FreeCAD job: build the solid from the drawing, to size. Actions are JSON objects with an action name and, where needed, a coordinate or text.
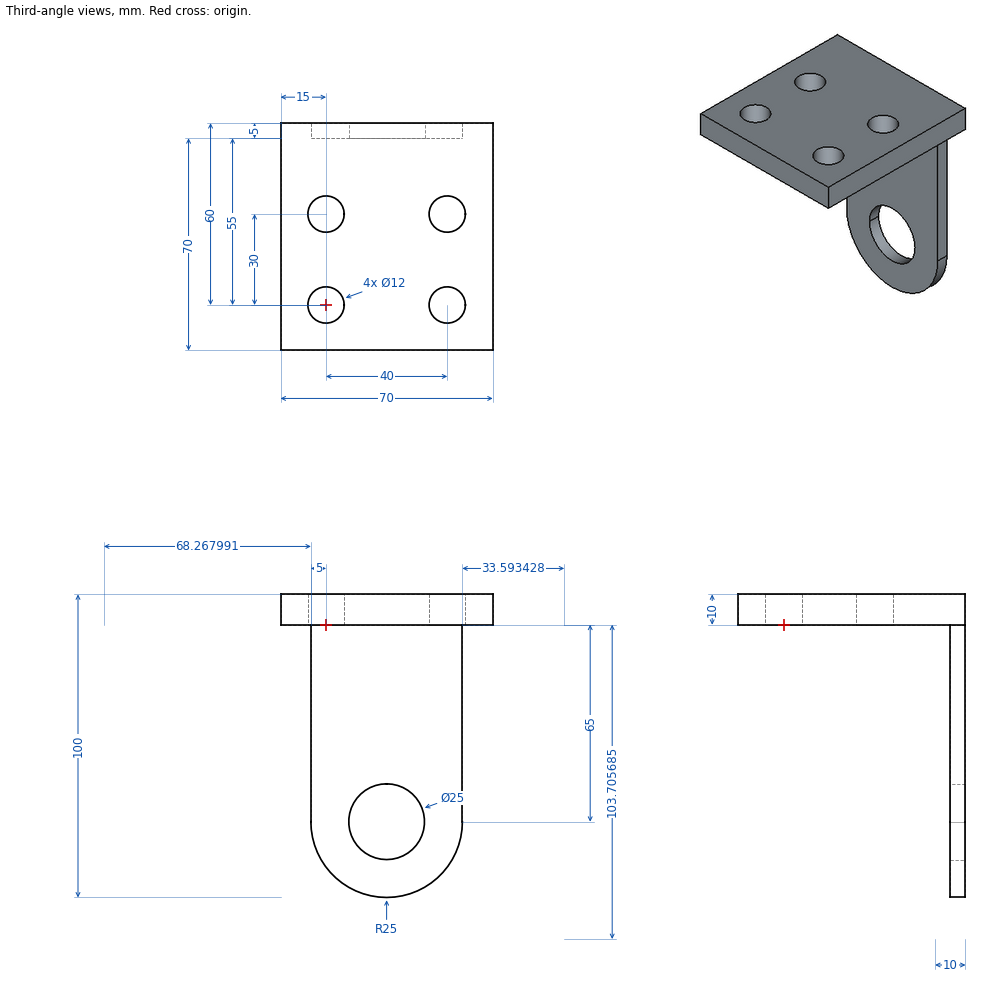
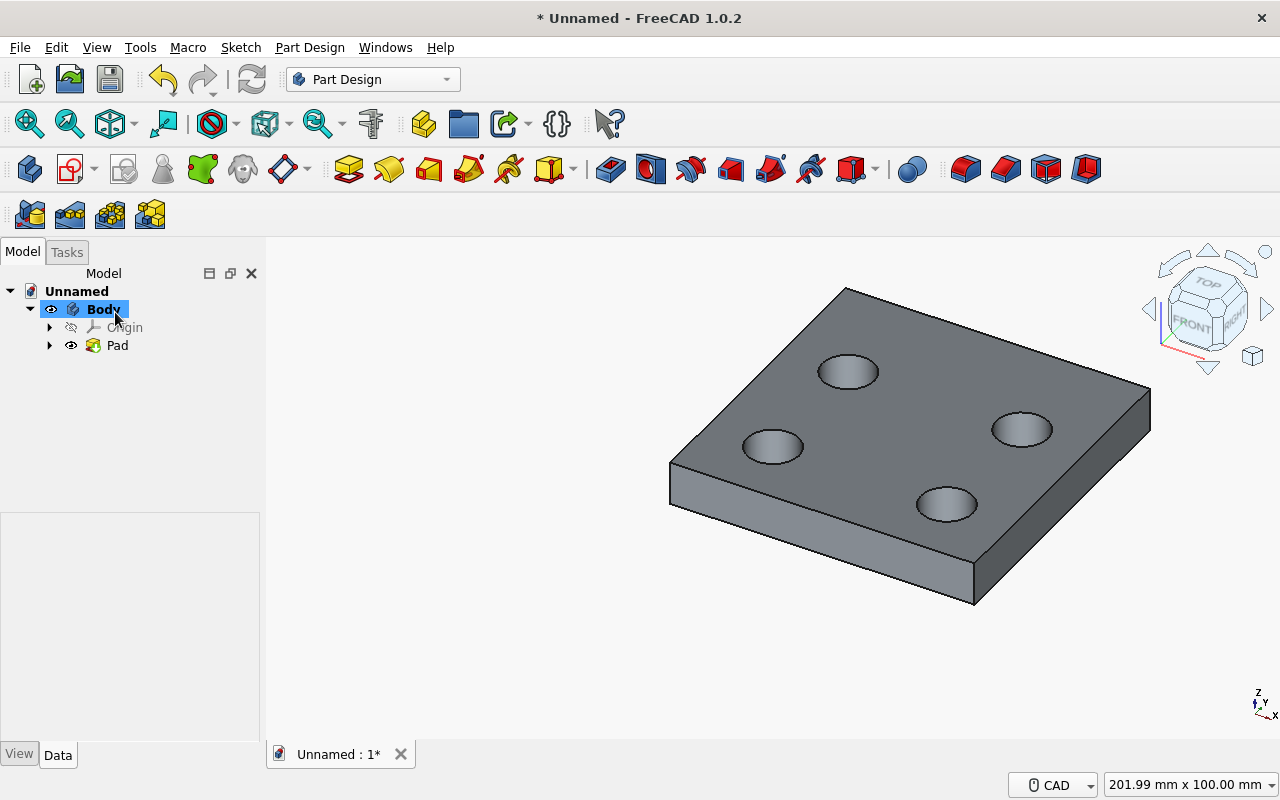
{"action": "left_click", "coordinate": [885, 450]}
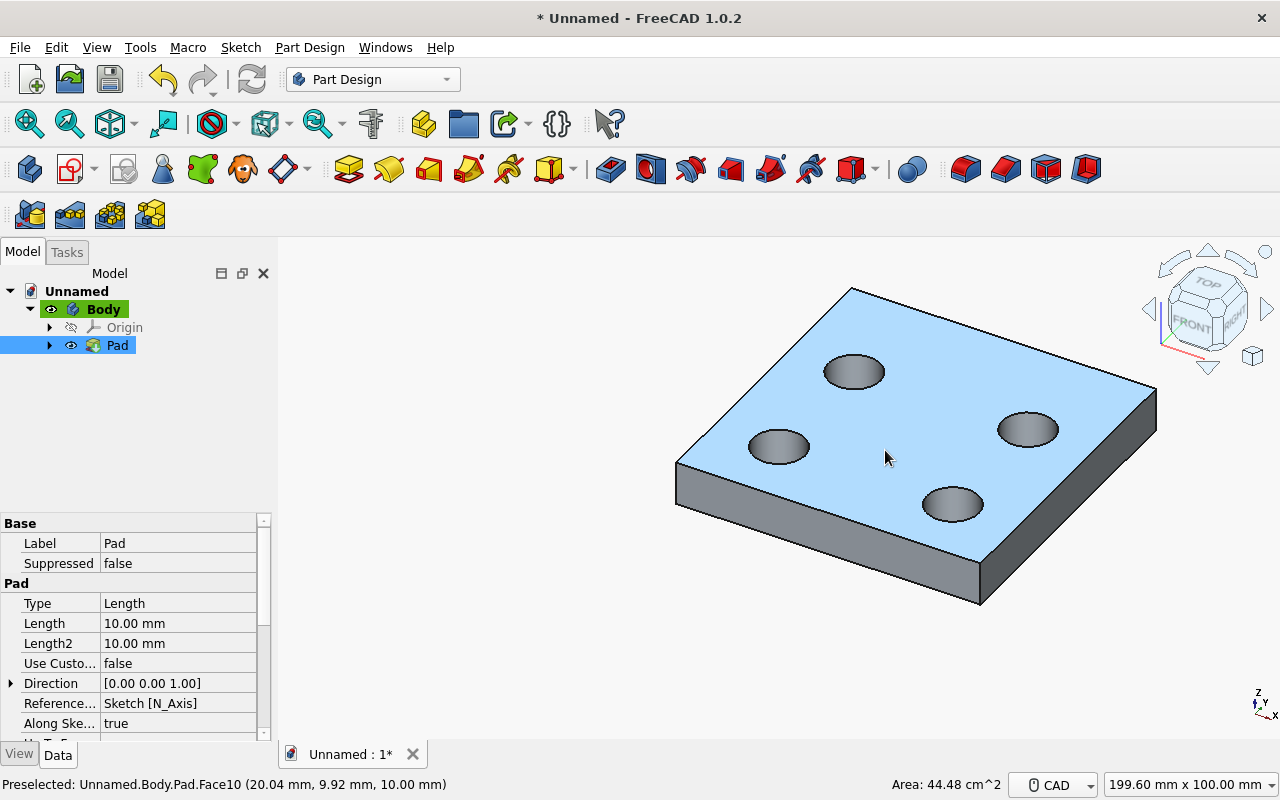
{"action": "left_click", "coordinate": [70, 170]}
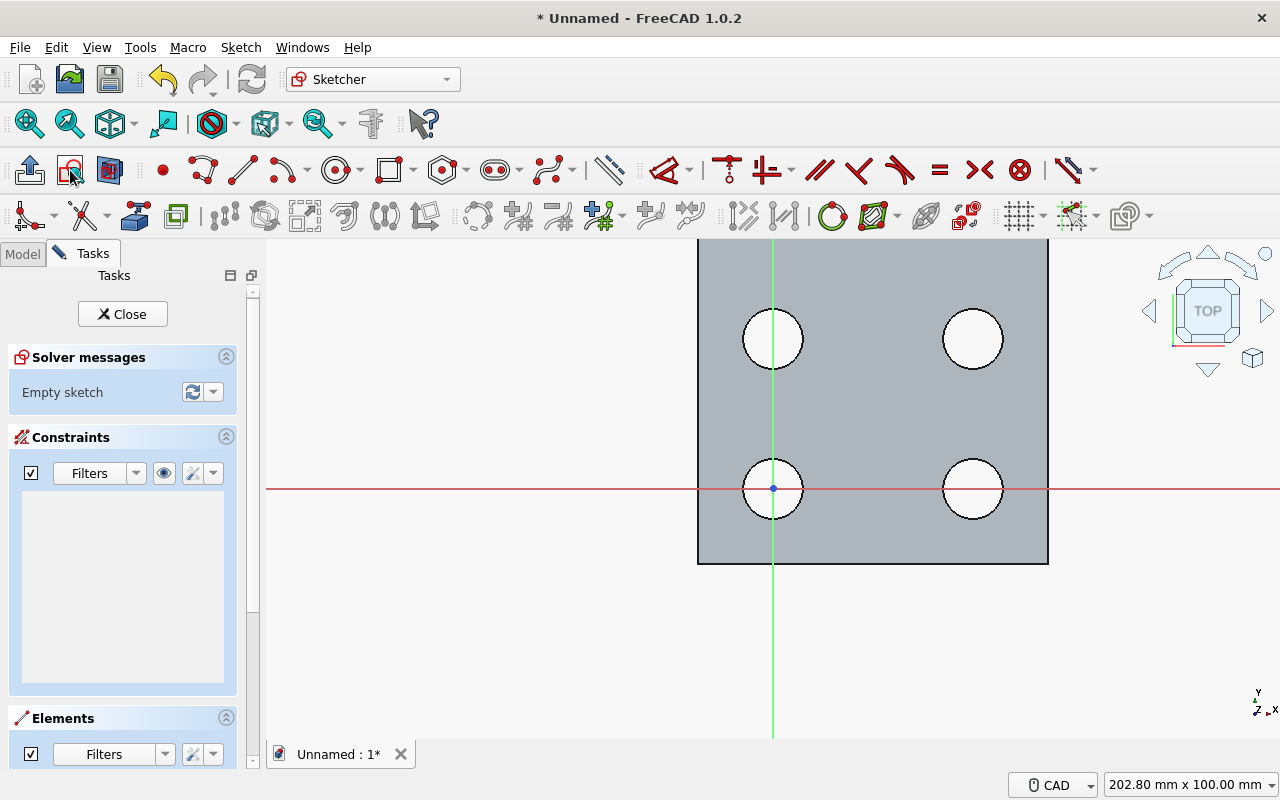
{"action": "scroll", "coordinate": [362, 711], "scroll_direction": "down", "scroll_amount": 2}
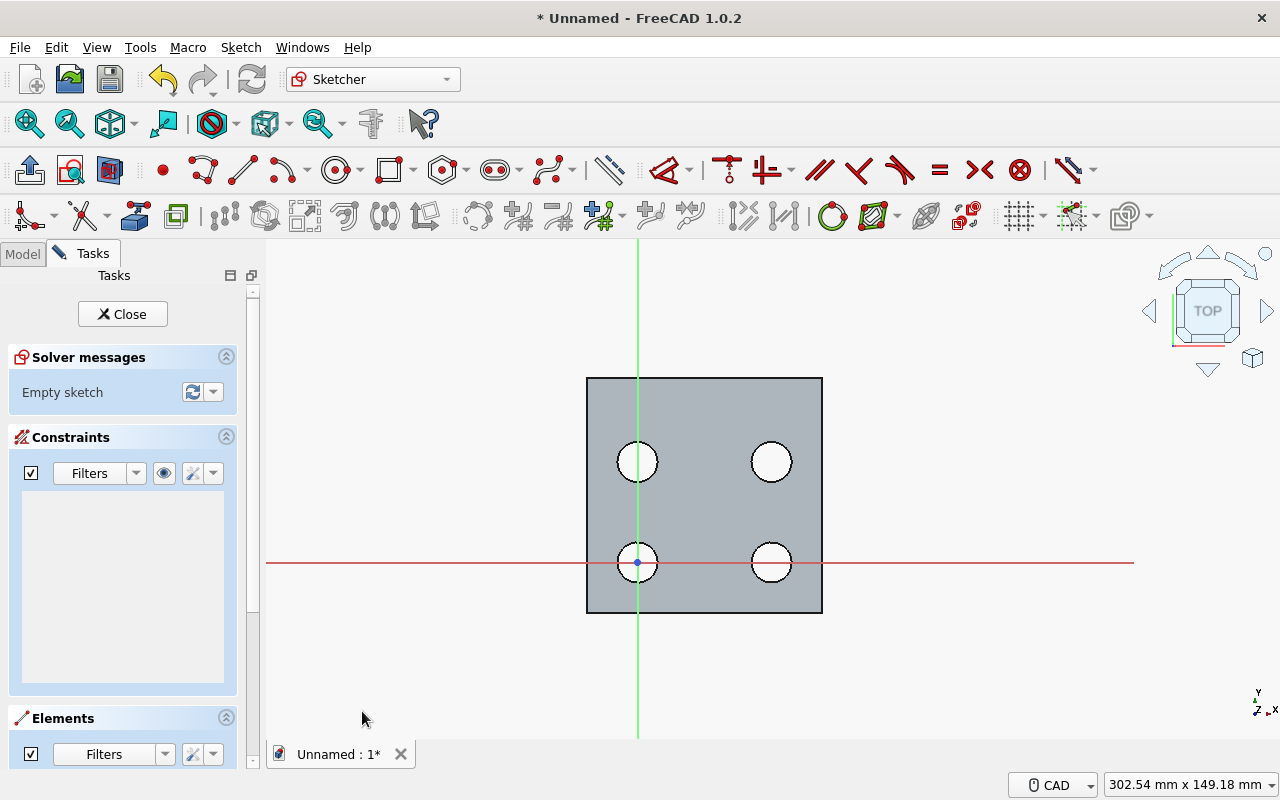
{"action": "scroll", "coordinate": [705, 407], "scroll_direction": "up", "scroll_amount": 2}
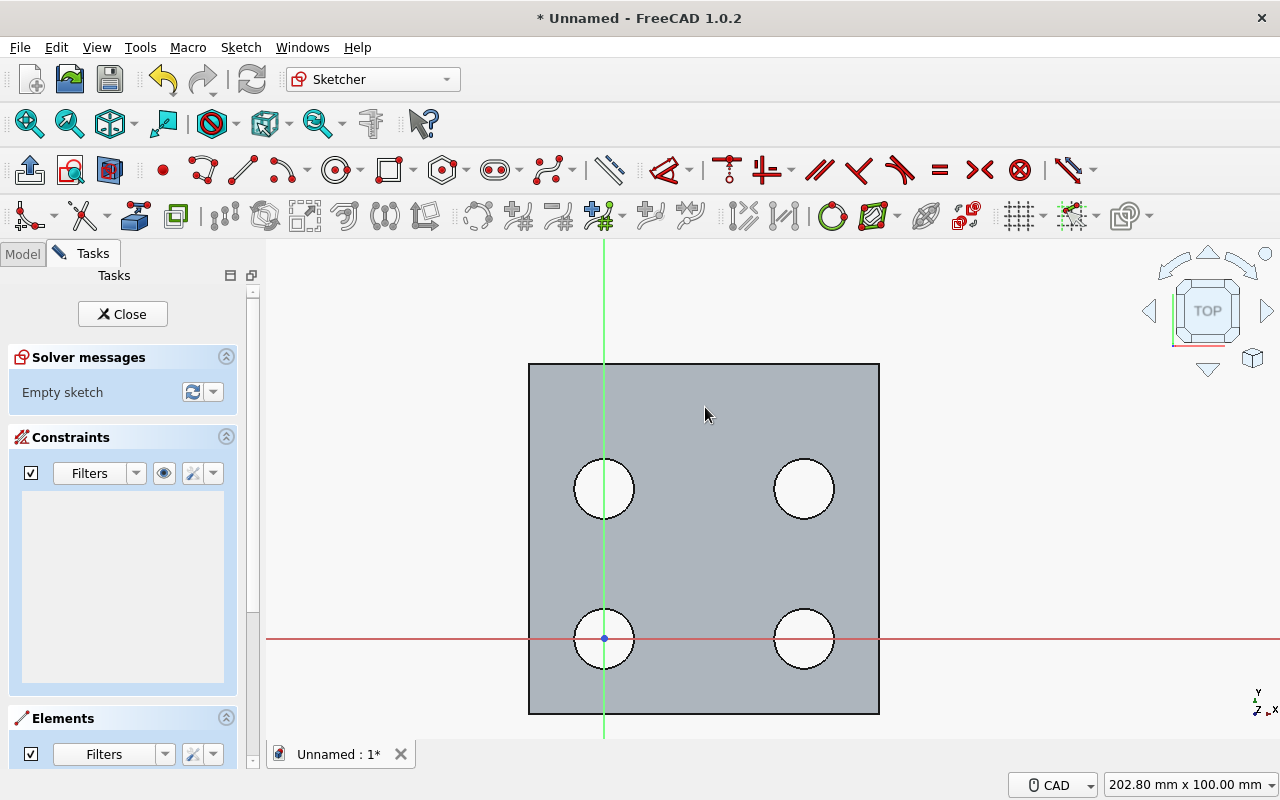
{"action": "left_click", "coordinate": [390, 170]}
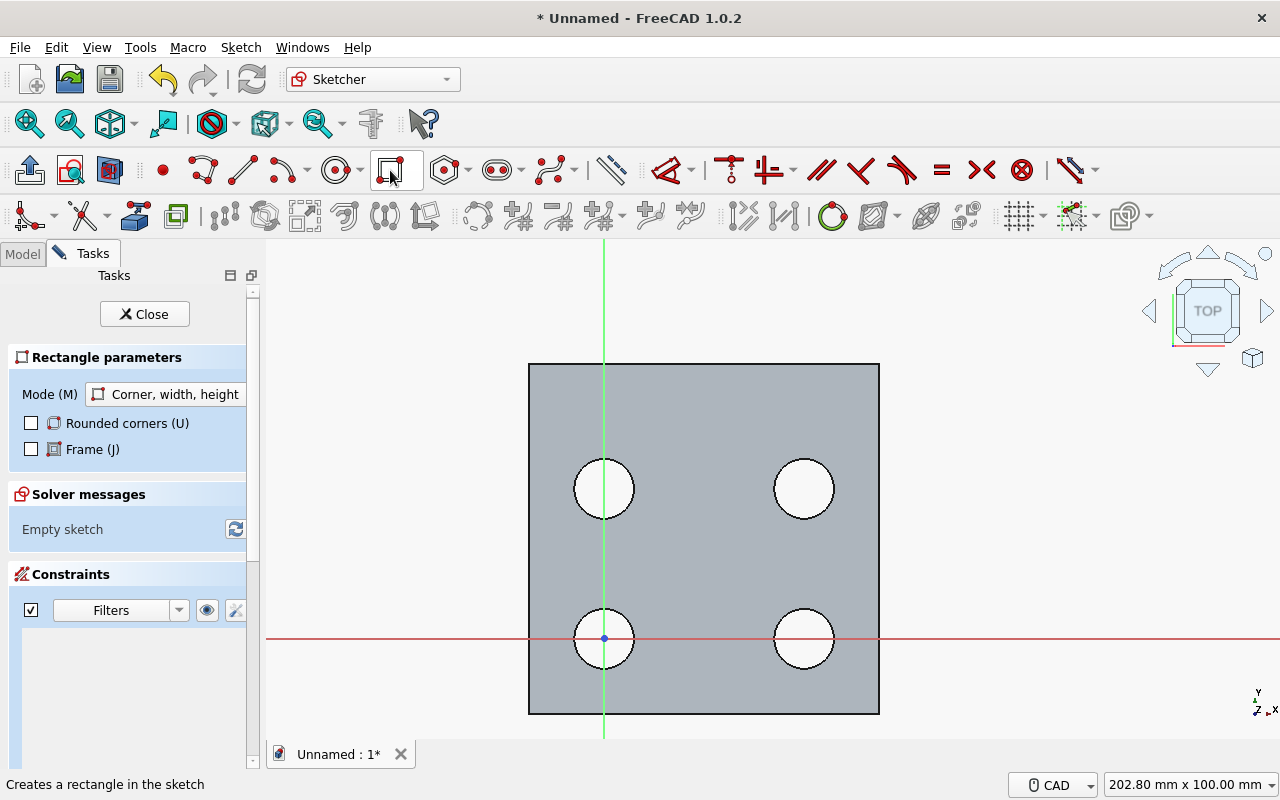
{"action": "left_click", "coordinate": [529, 339]}
{"action": "left_click", "coordinate": [879, 364]}
{"action": "key", "text": "Escape"}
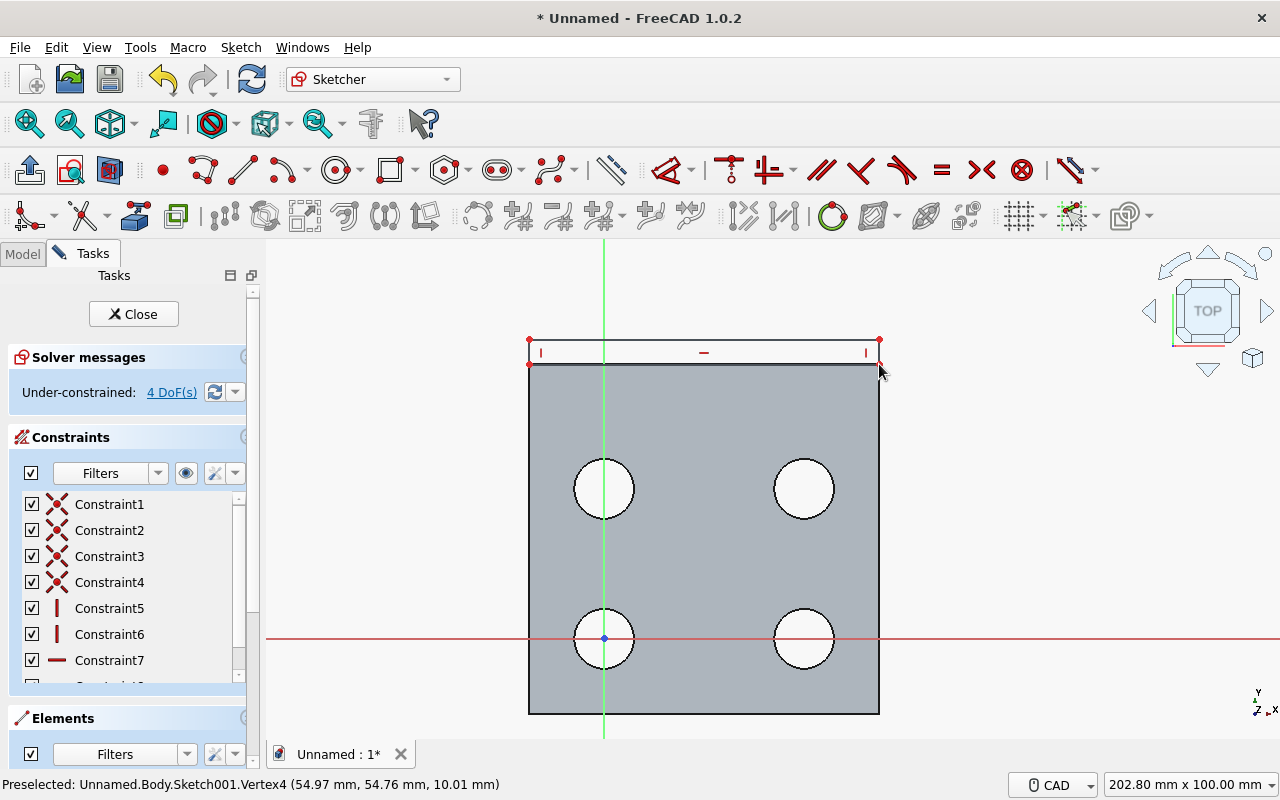
{"action": "left_click", "coordinate": [666, 170]}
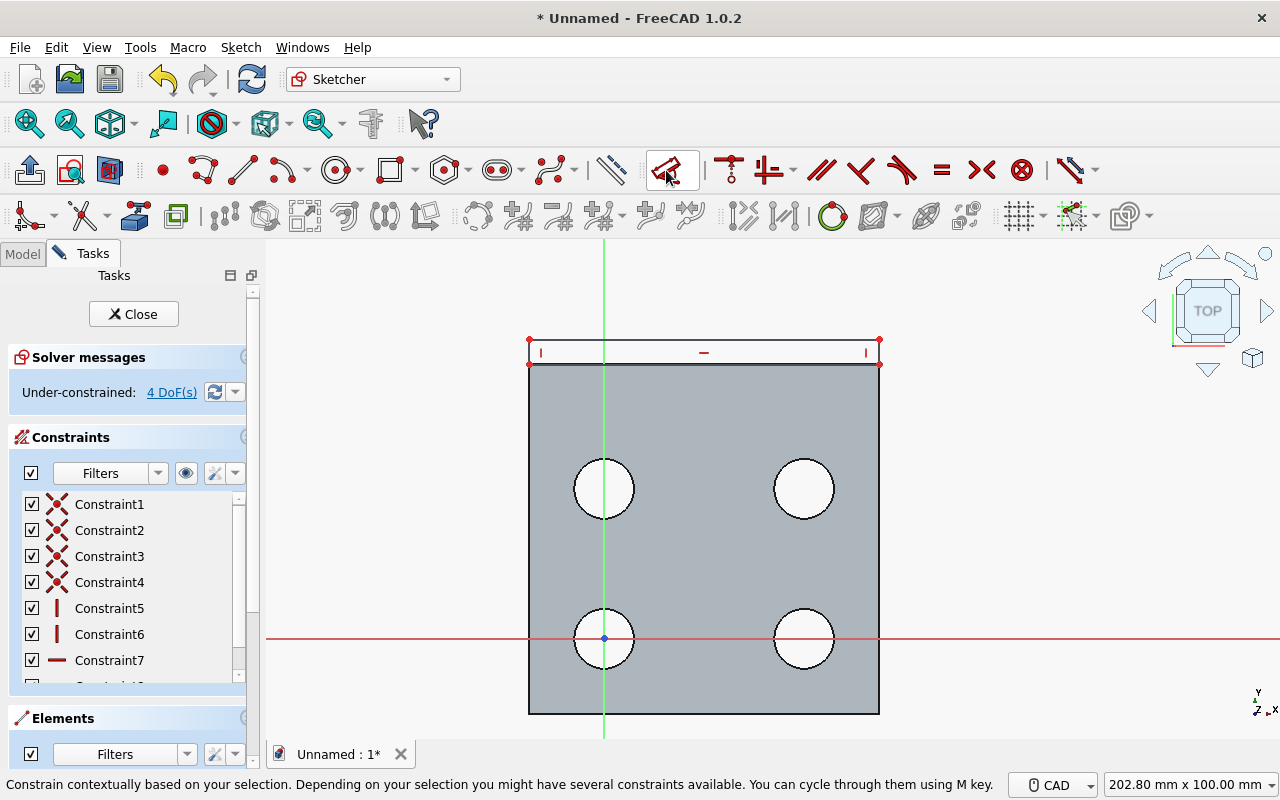
{"action": "scroll", "coordinate": [529, 350], "scroll_direction": "up", "scroll_amount": 3}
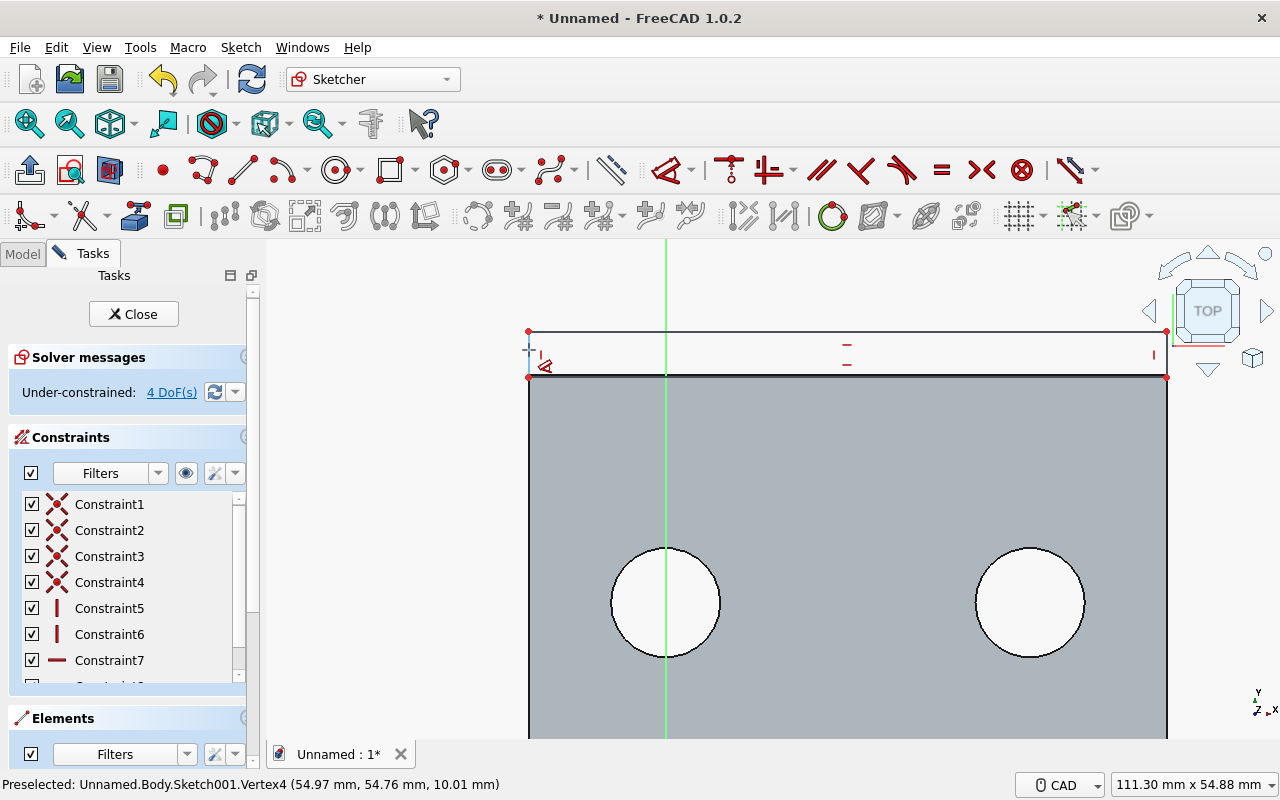
{"action": "left_click", "coordinate": [529, 350]}
{"action": "left_click", "coordinate": [495, 354]}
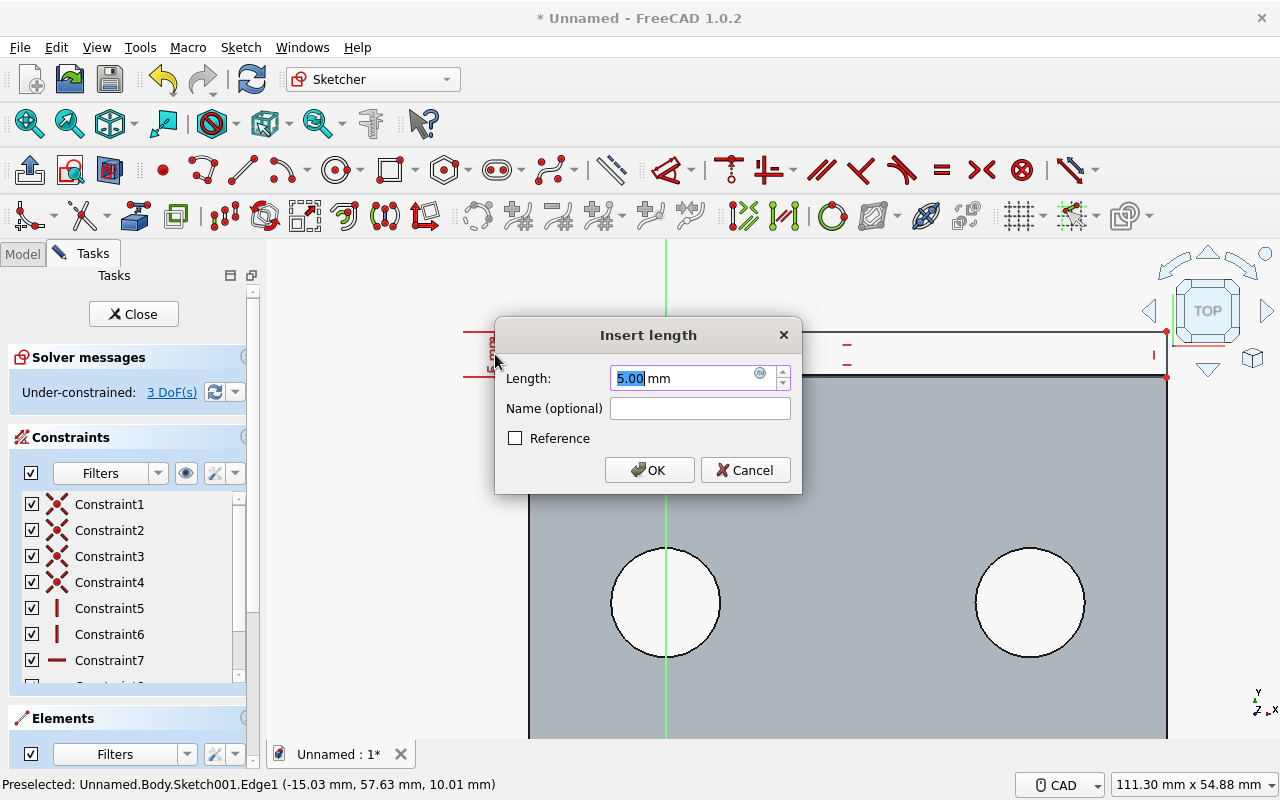
{"action": "type", "text": "5"}
{"action": "key", "text": "Return"}